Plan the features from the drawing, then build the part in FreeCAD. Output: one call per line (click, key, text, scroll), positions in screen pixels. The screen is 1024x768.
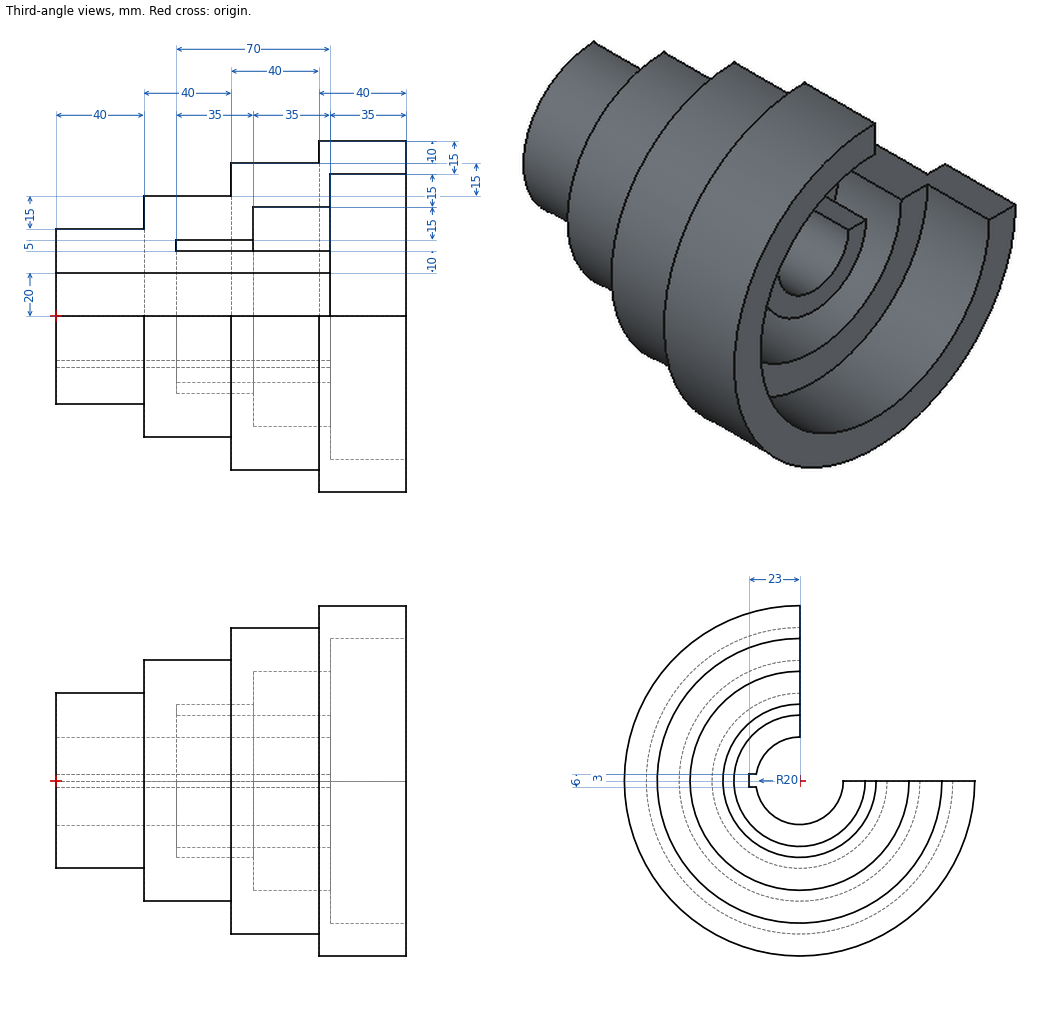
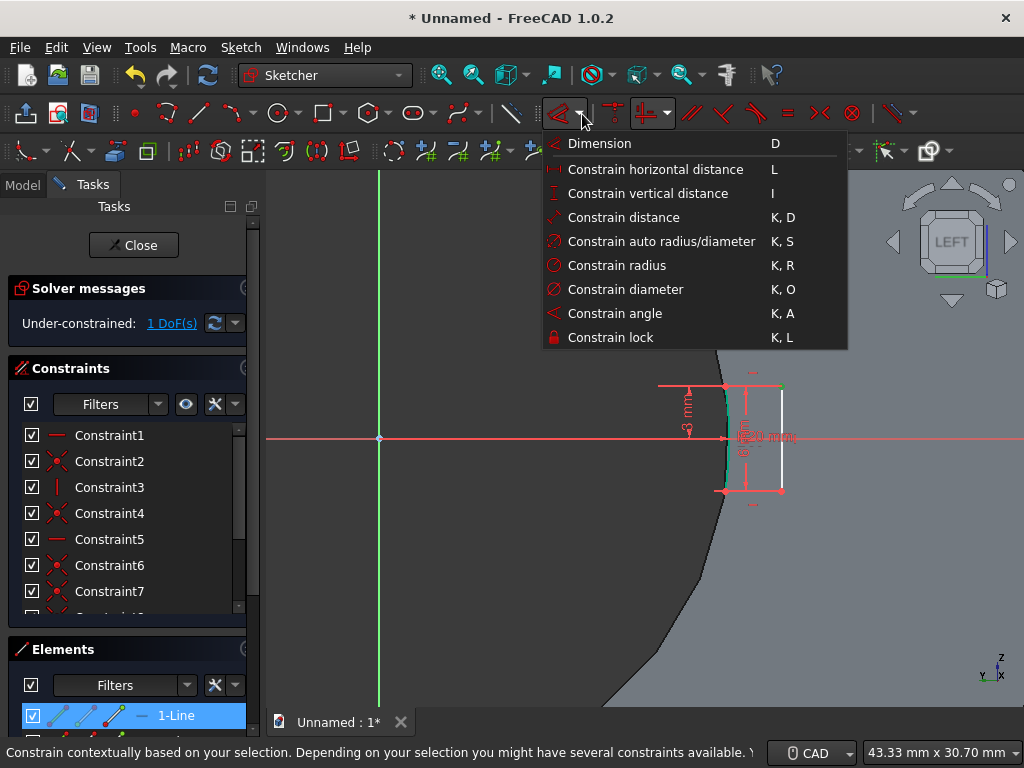
click(695, 169)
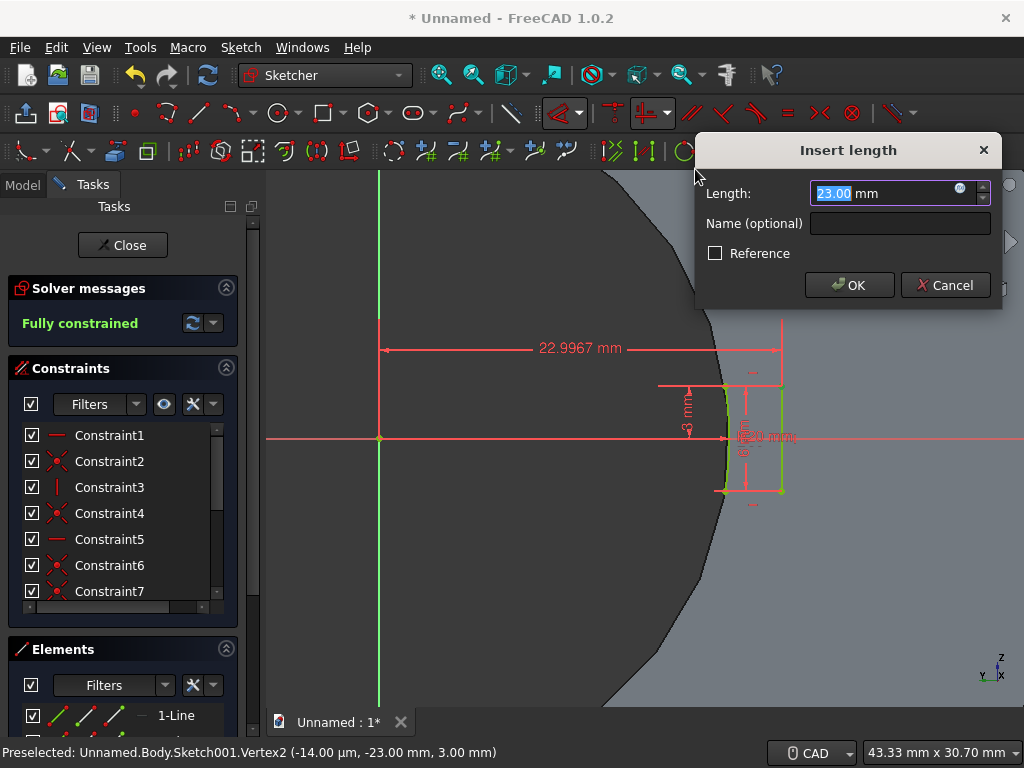
text(23)
key(Return)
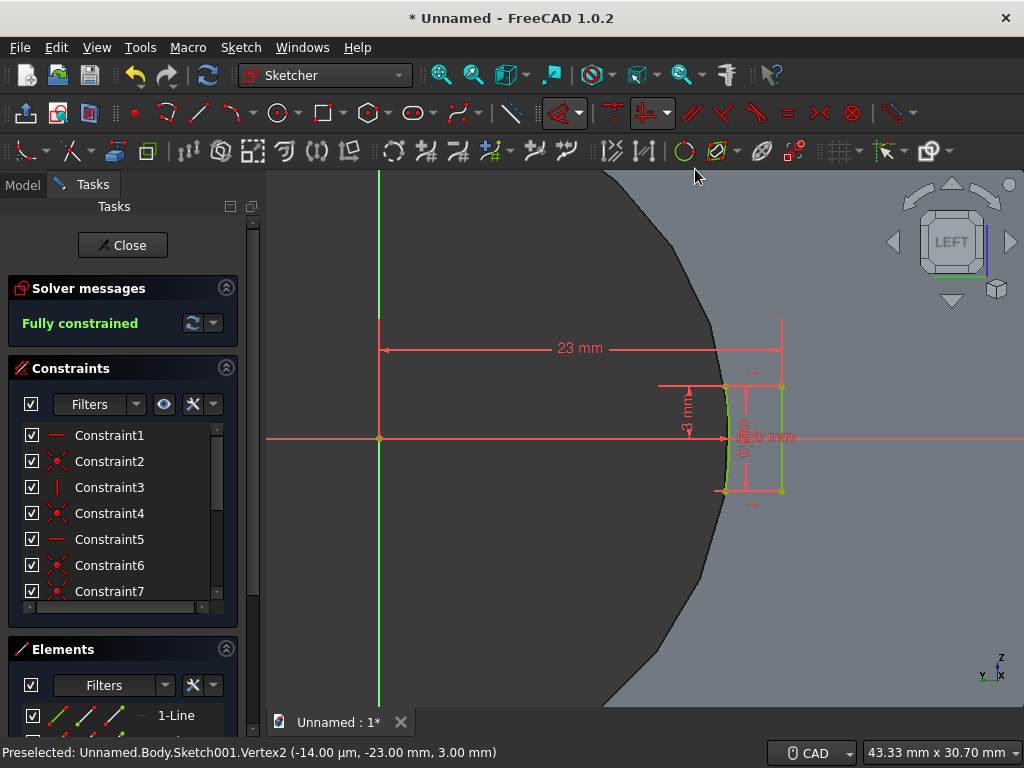
click(123, 245)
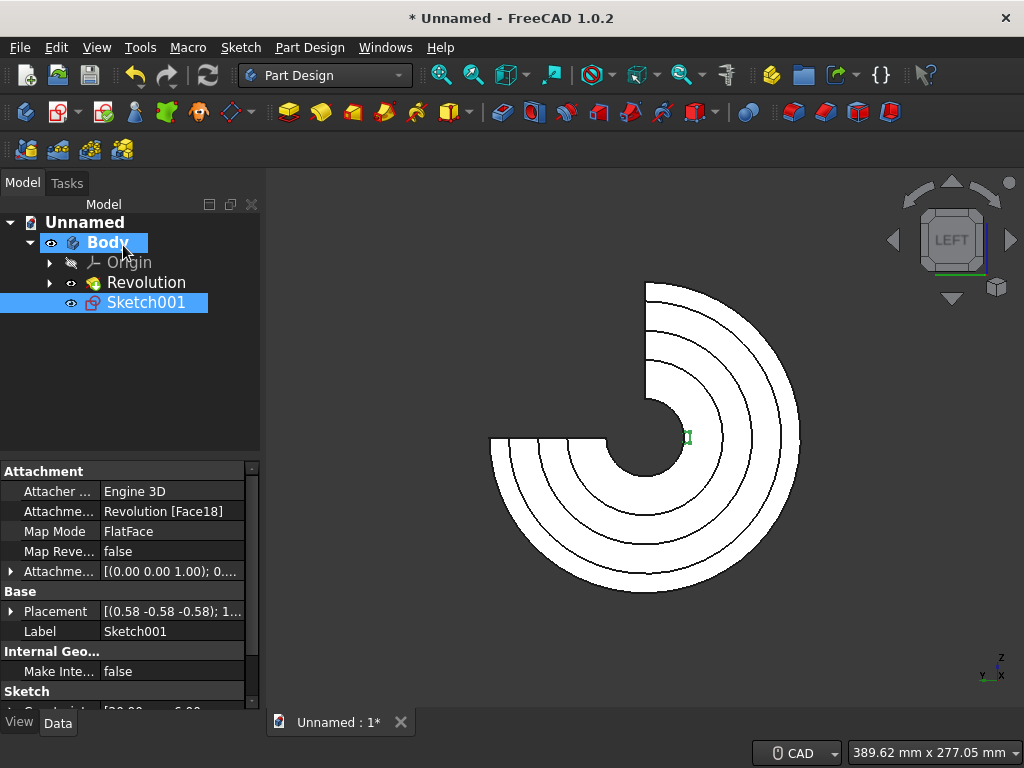
click(504, 112)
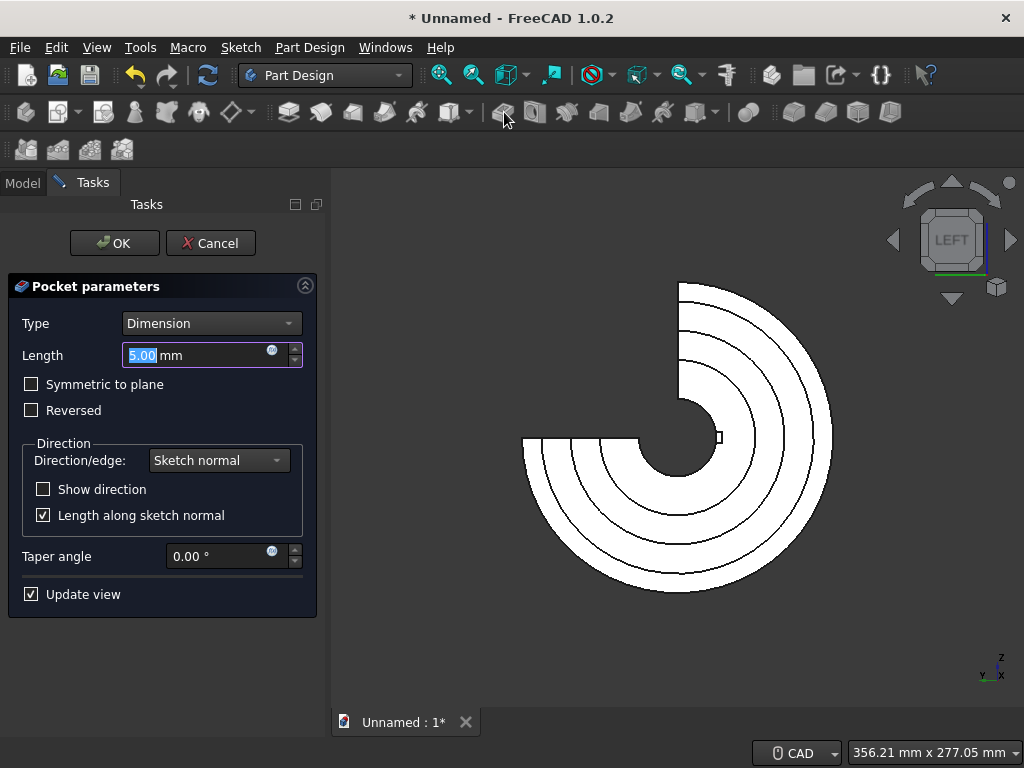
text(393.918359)
key(Tab)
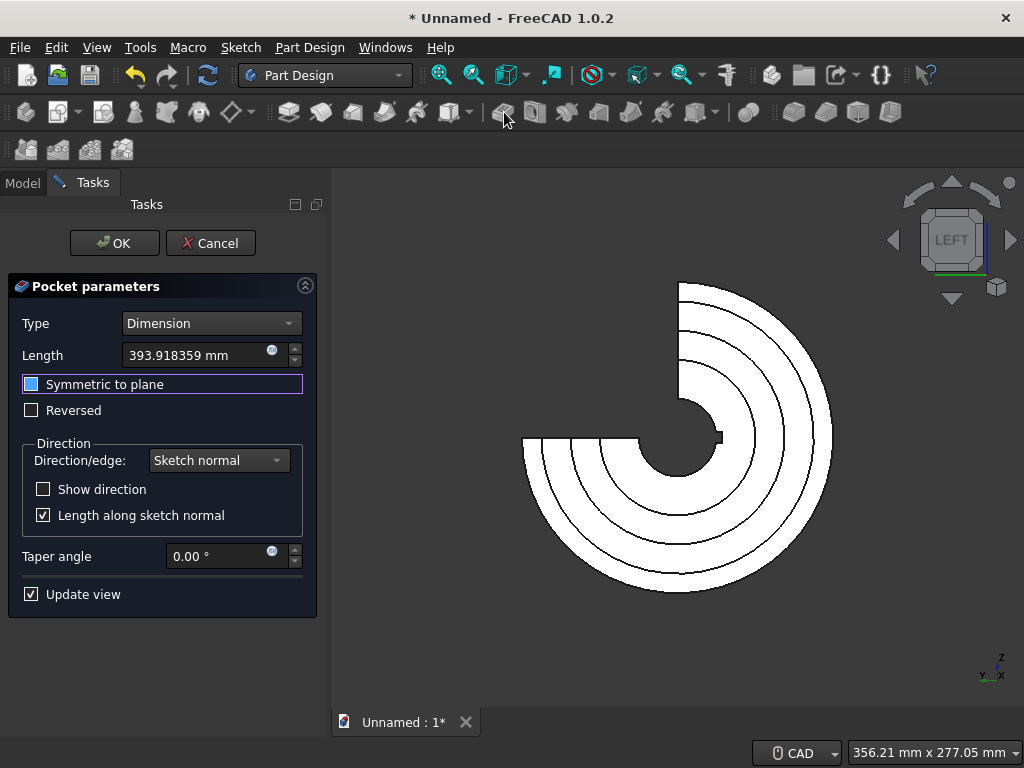
click(30, 384)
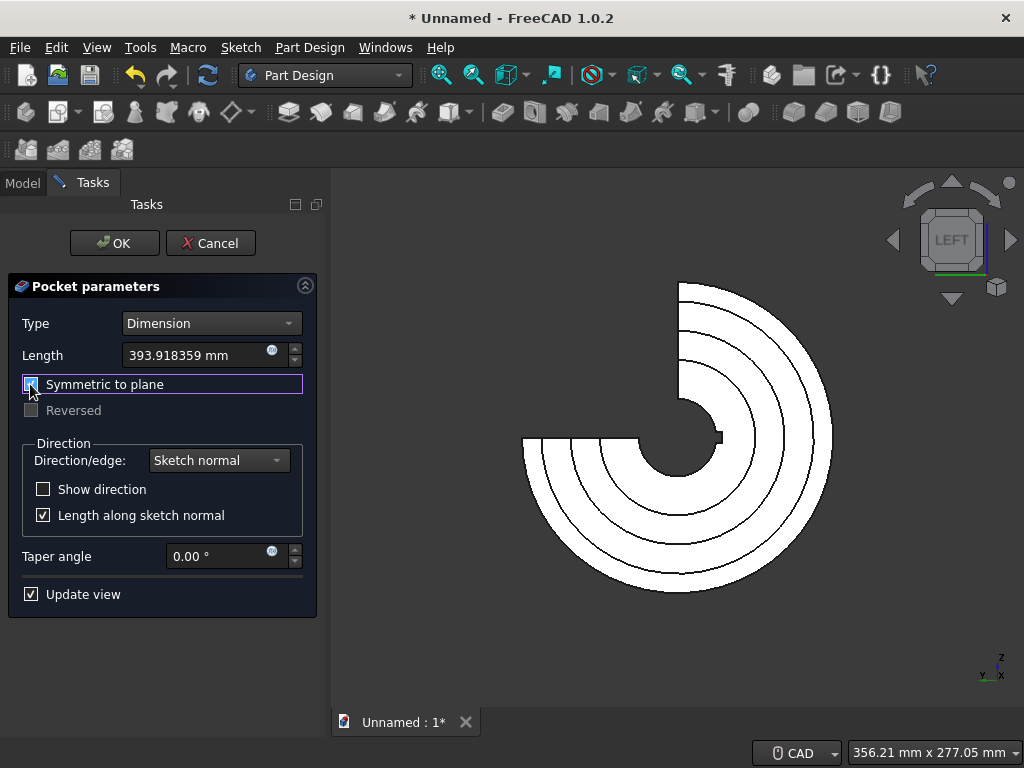
click(115, 243)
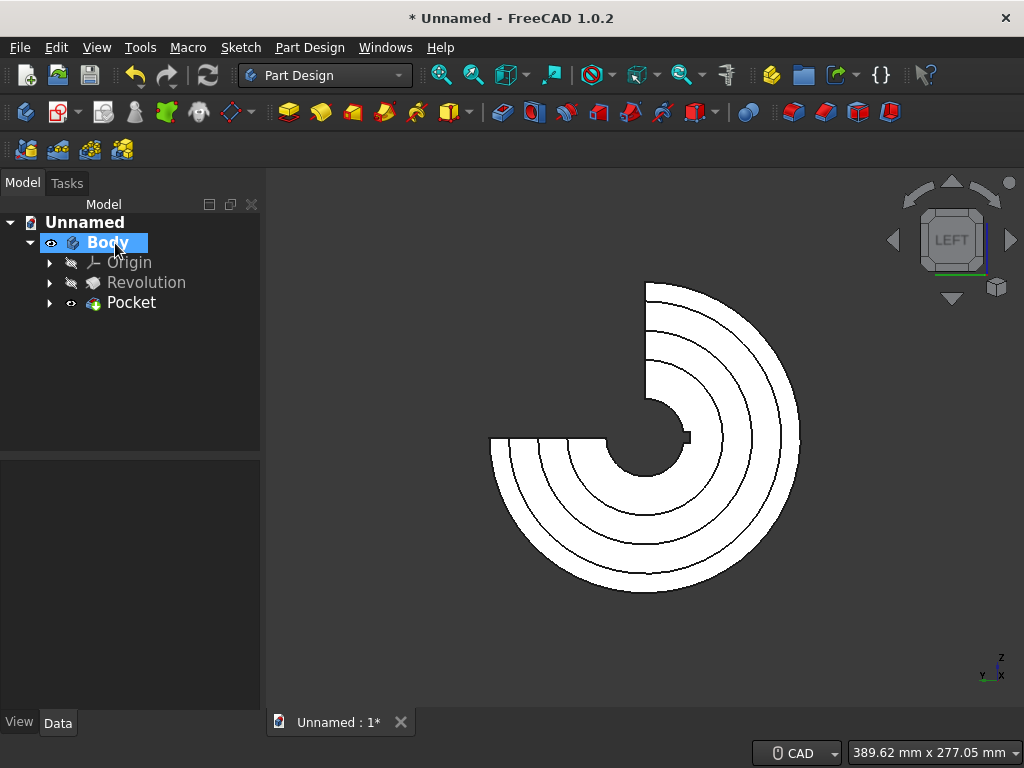
key(0)